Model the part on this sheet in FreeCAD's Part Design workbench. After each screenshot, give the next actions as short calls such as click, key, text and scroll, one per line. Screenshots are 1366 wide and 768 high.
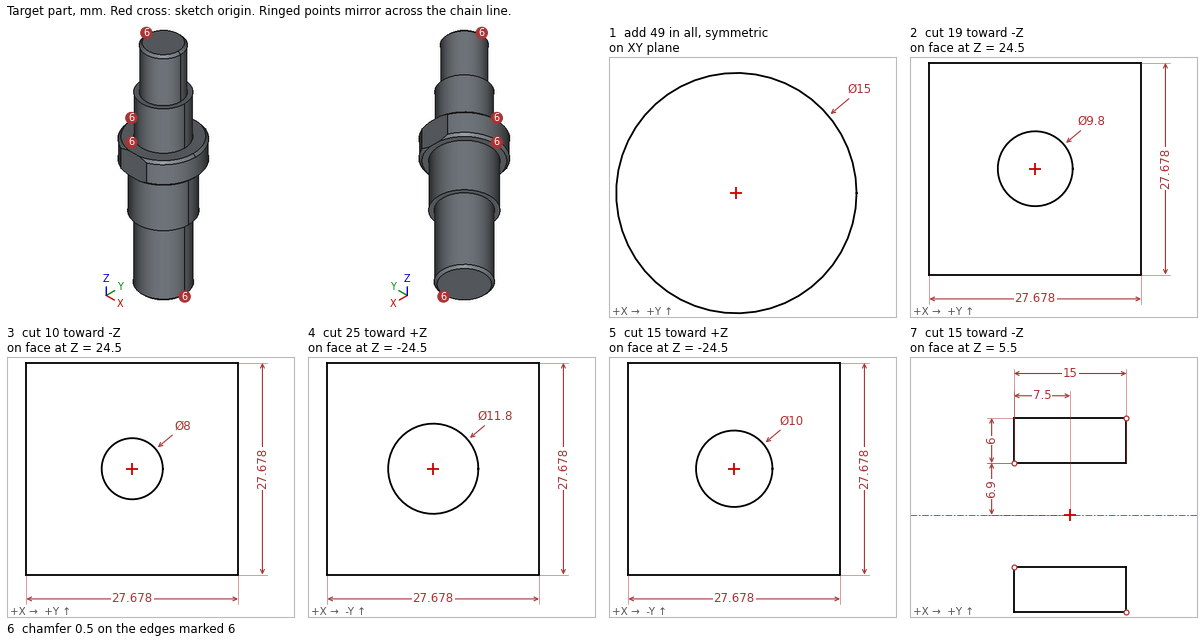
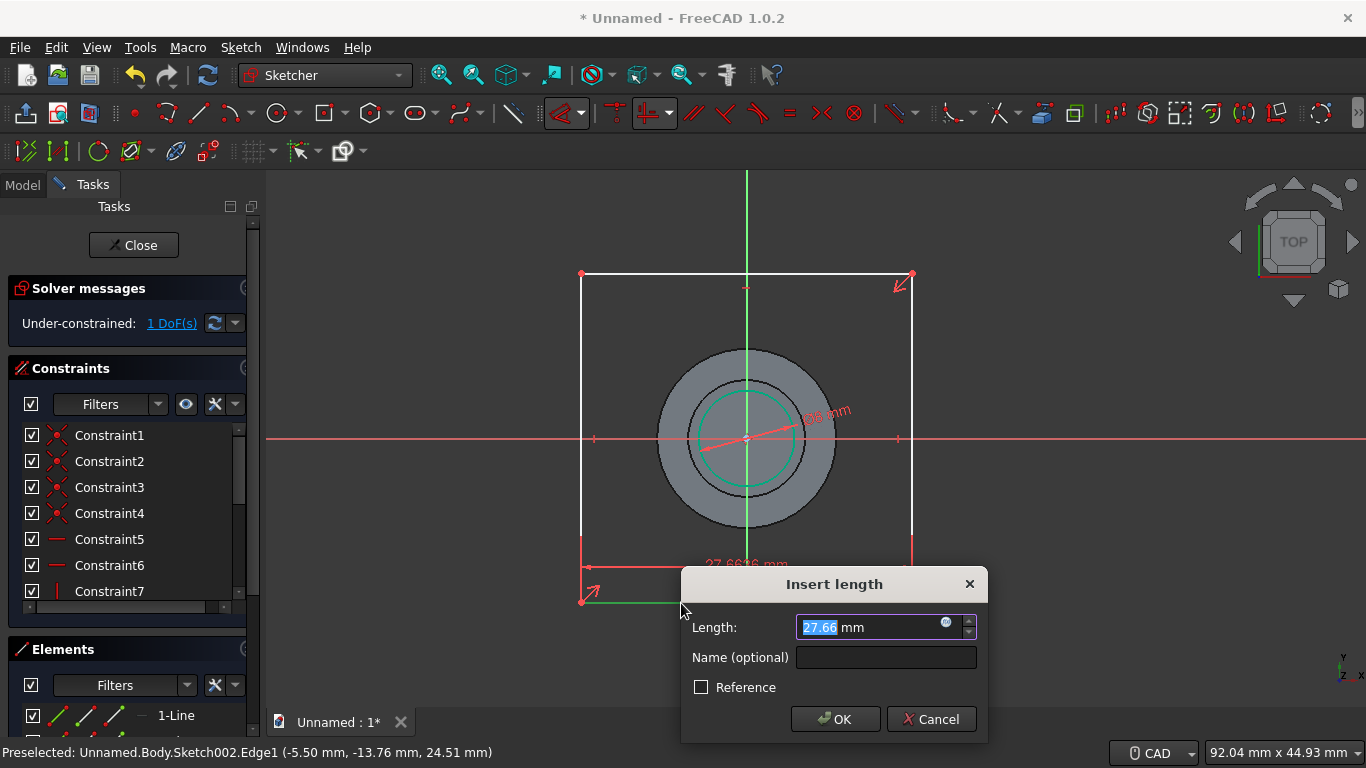
text(27.678)
key(Return)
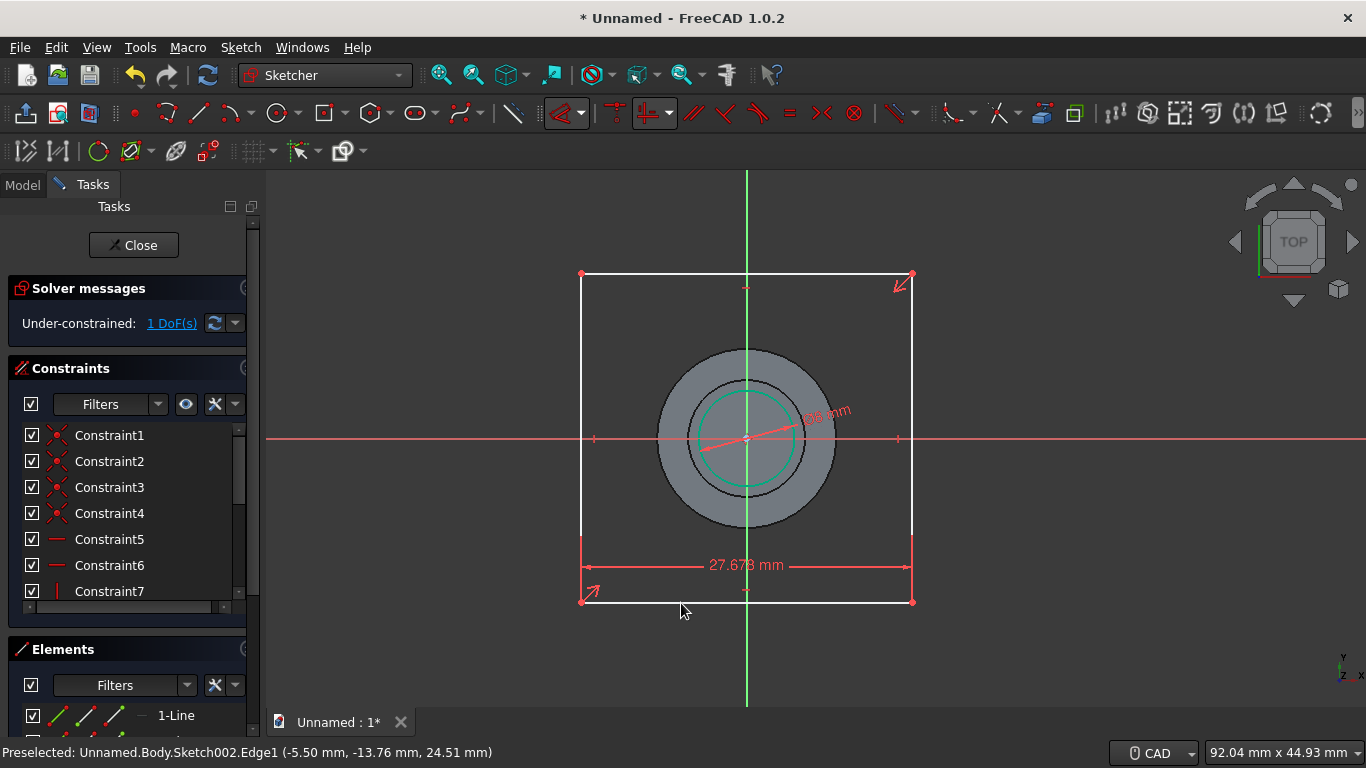
click(912, 504)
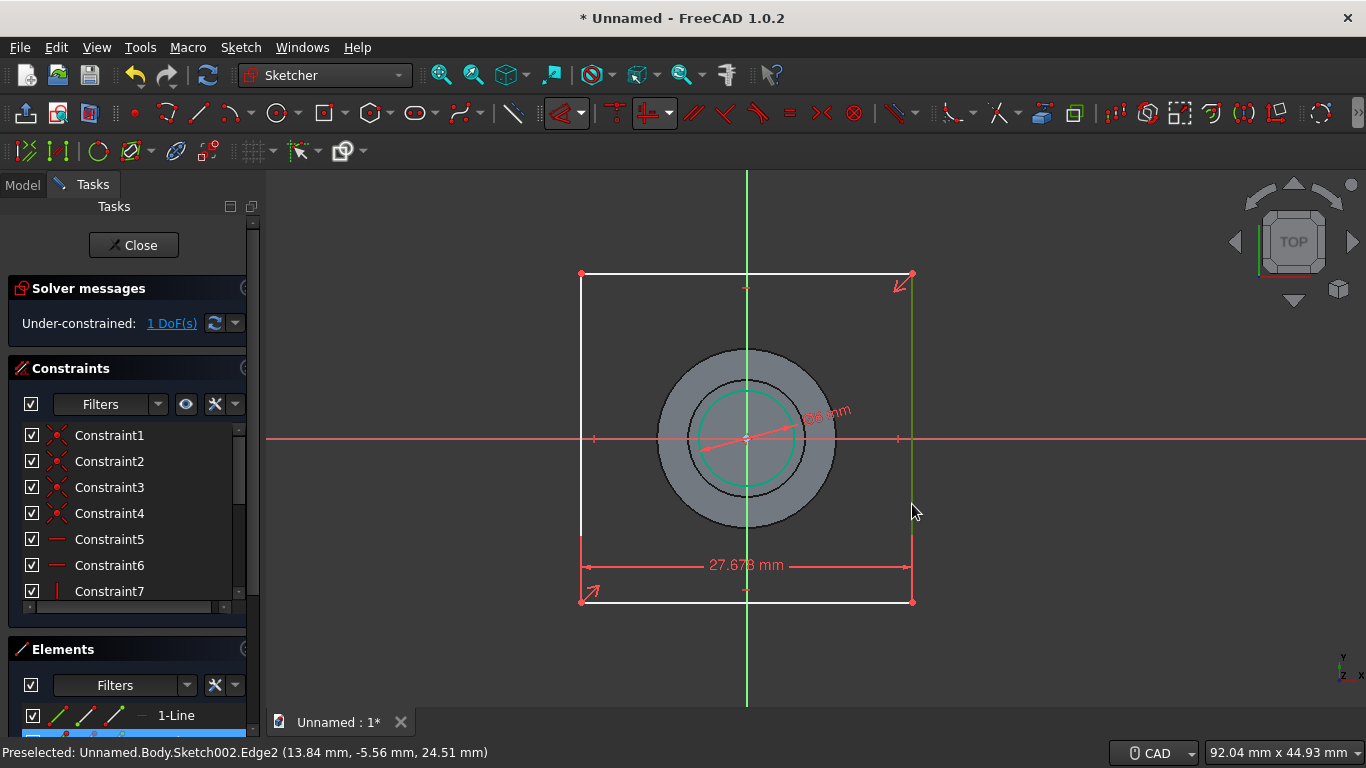
key(i)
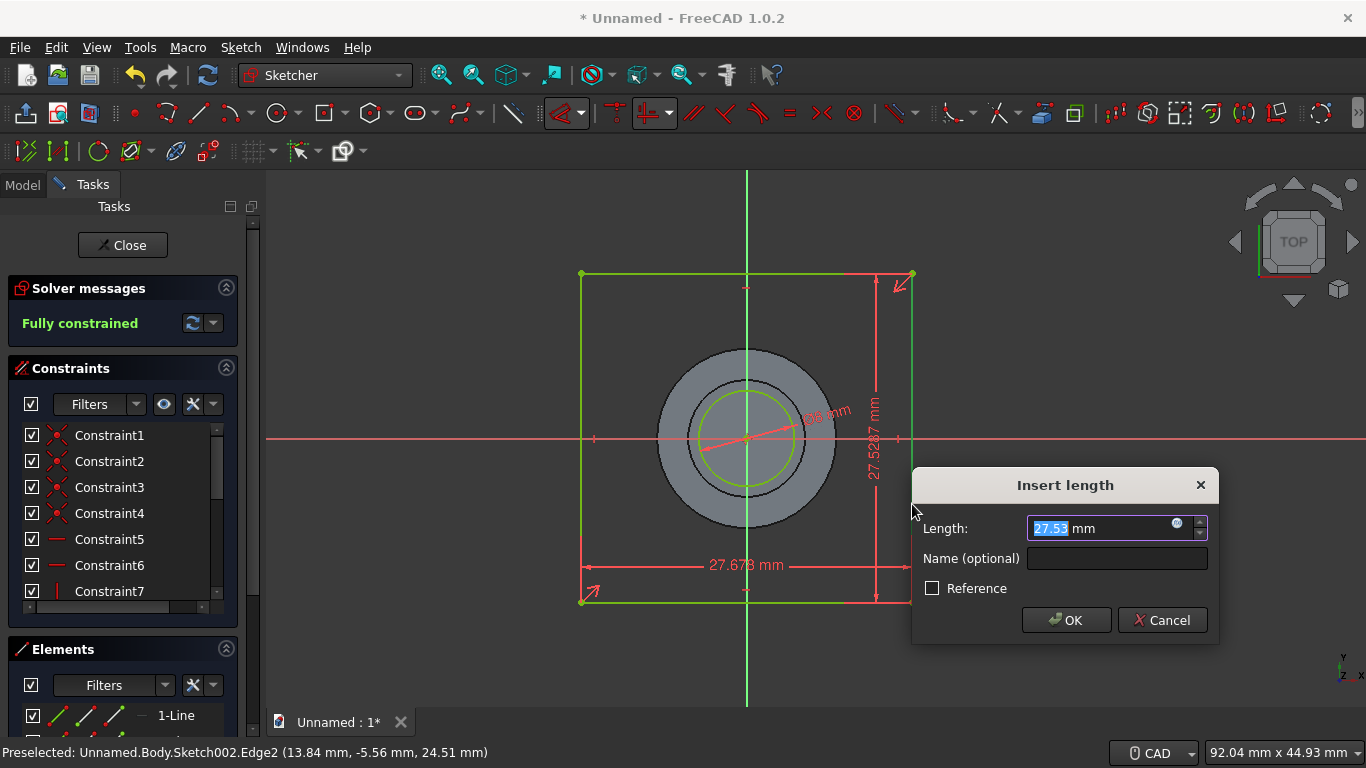
text(27.678)
key(Return)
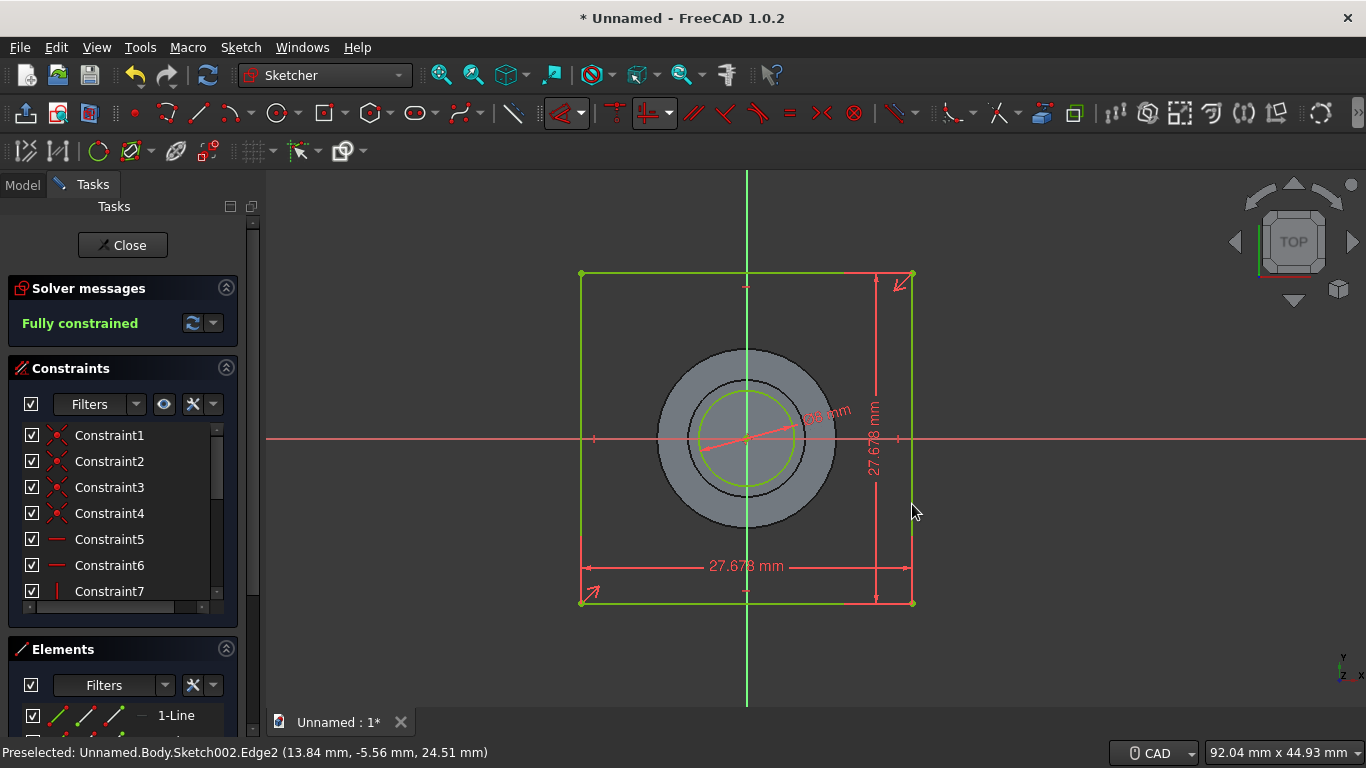
click(123, 245)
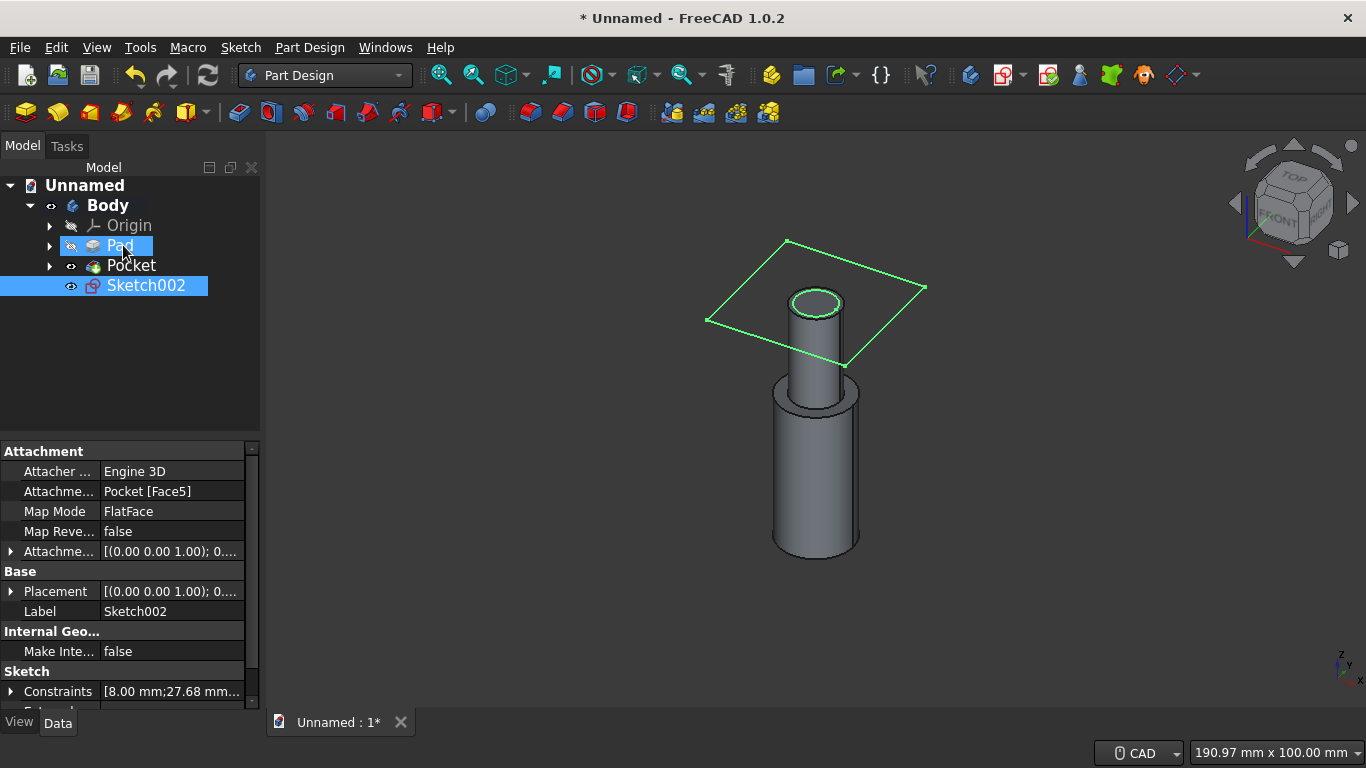
click(240, 112)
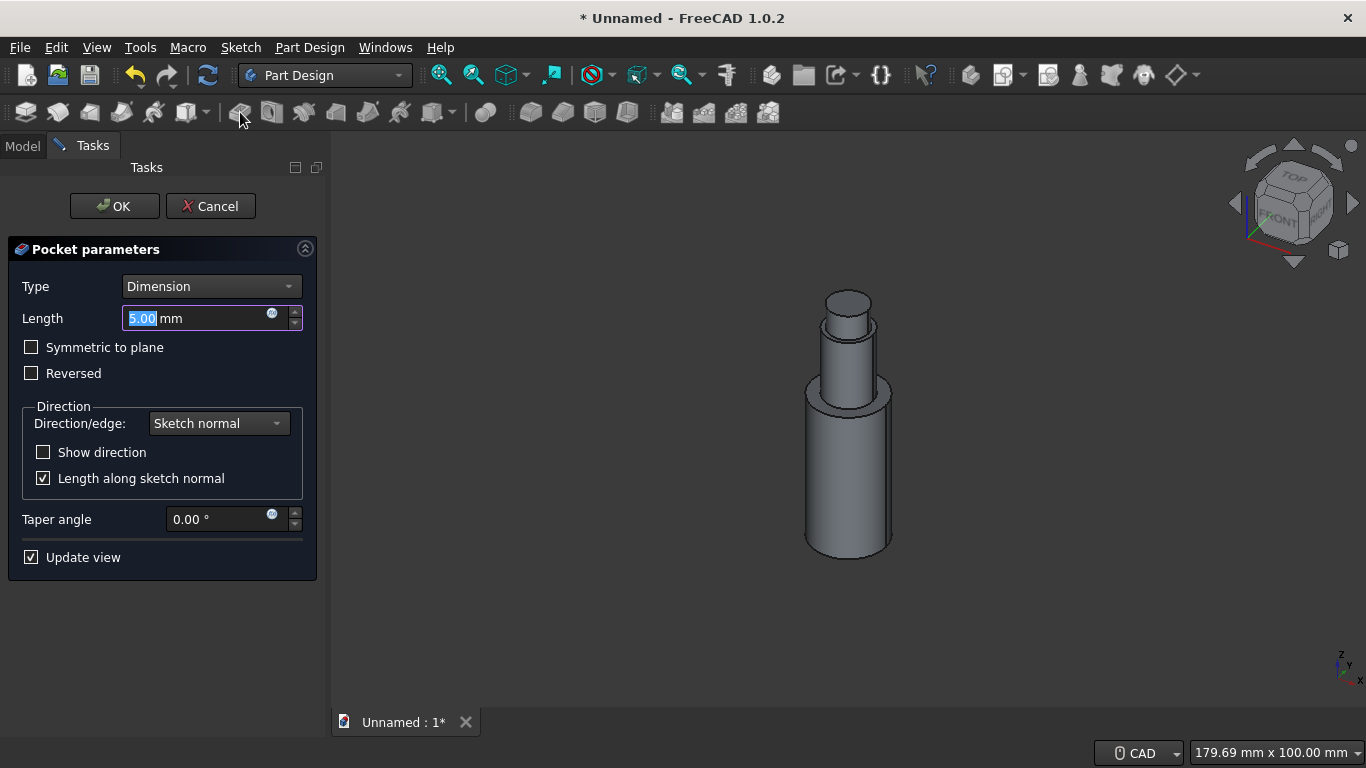
text(10)
key(Tab)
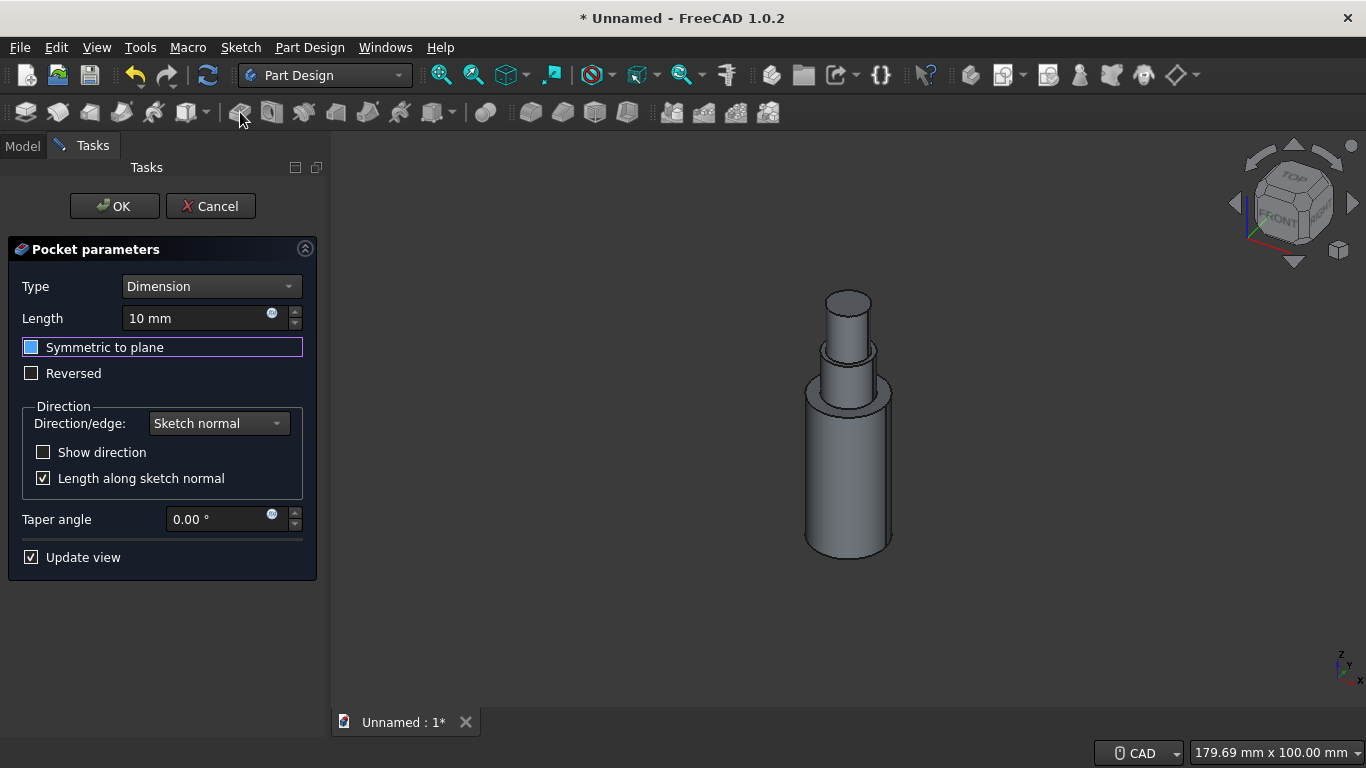
click(115, 206)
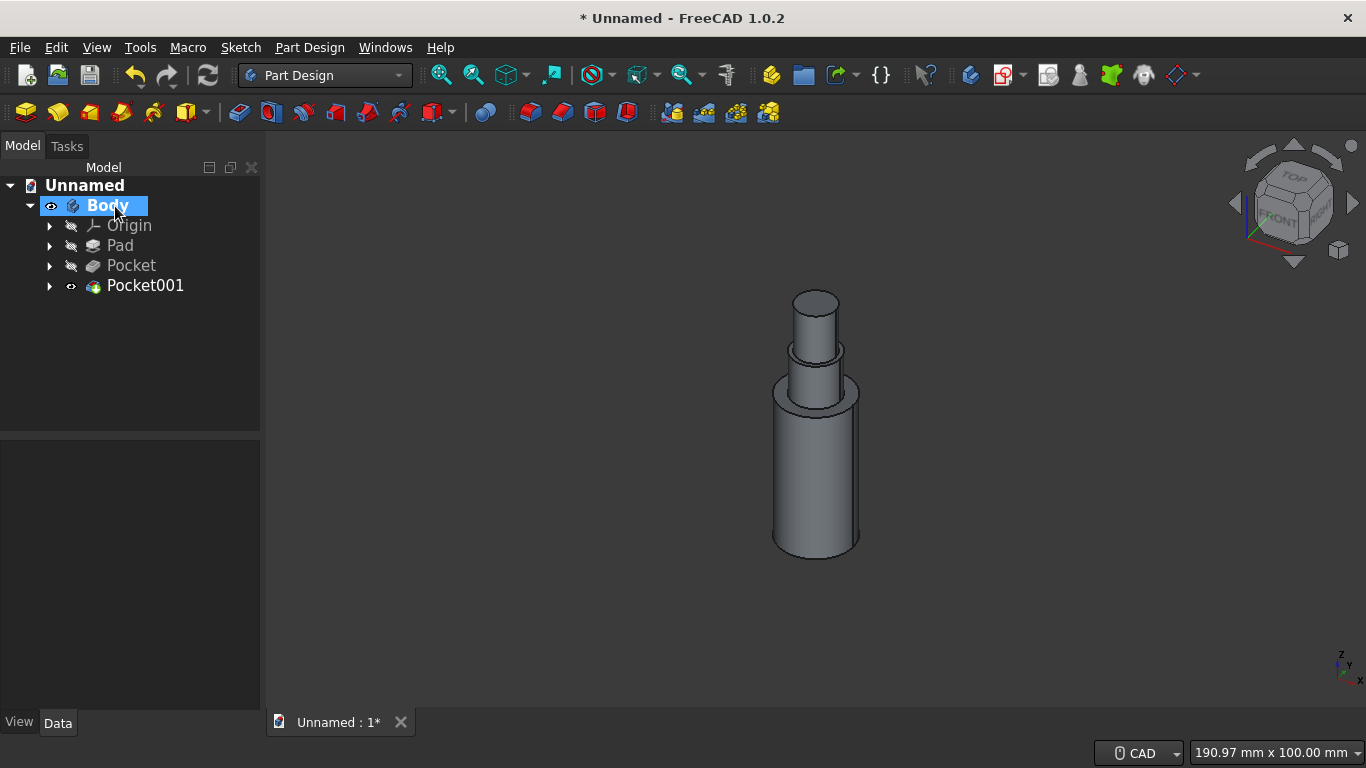
key(5)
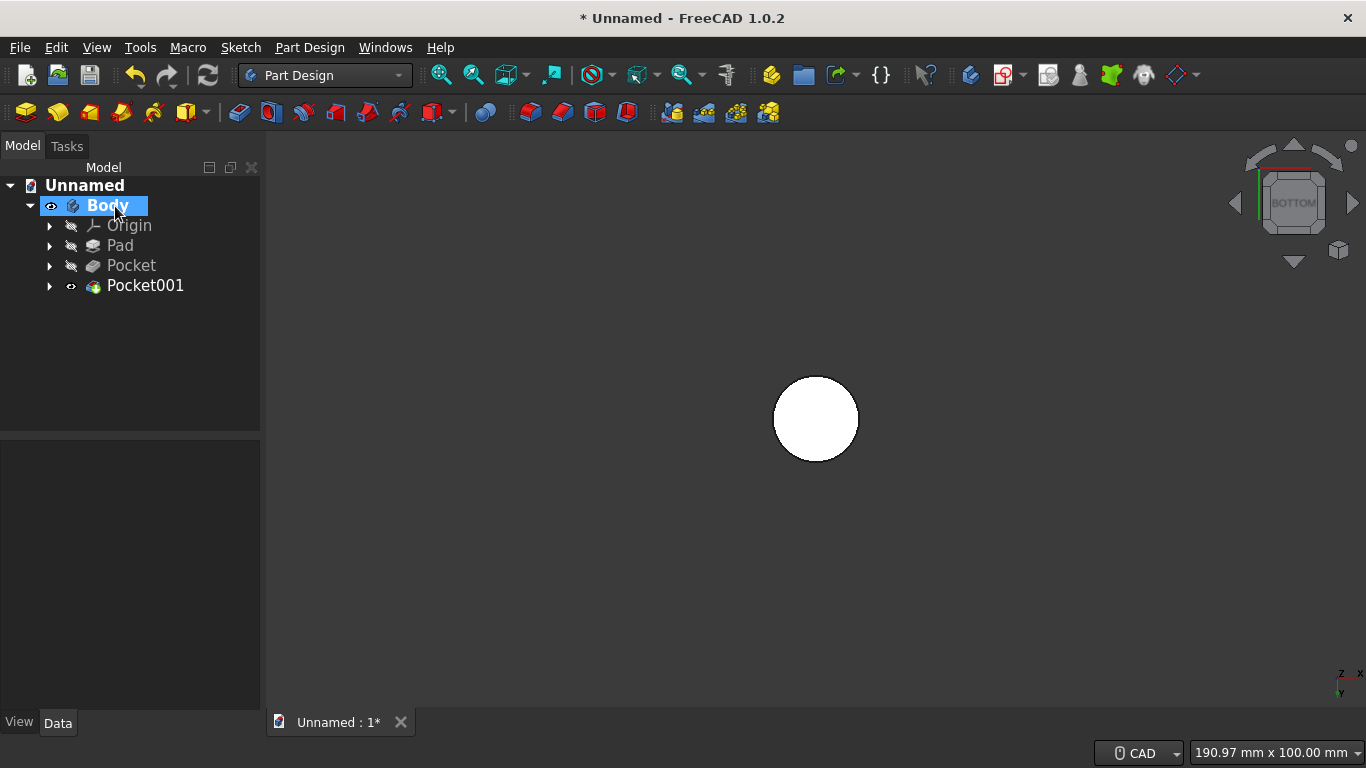
click(442, 76)